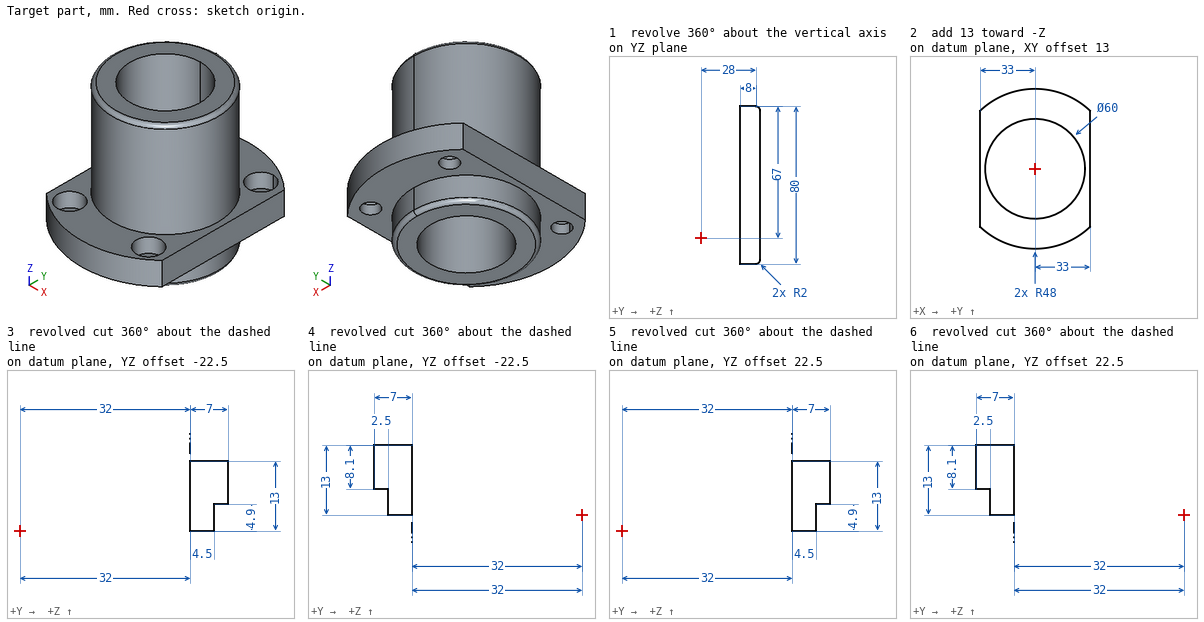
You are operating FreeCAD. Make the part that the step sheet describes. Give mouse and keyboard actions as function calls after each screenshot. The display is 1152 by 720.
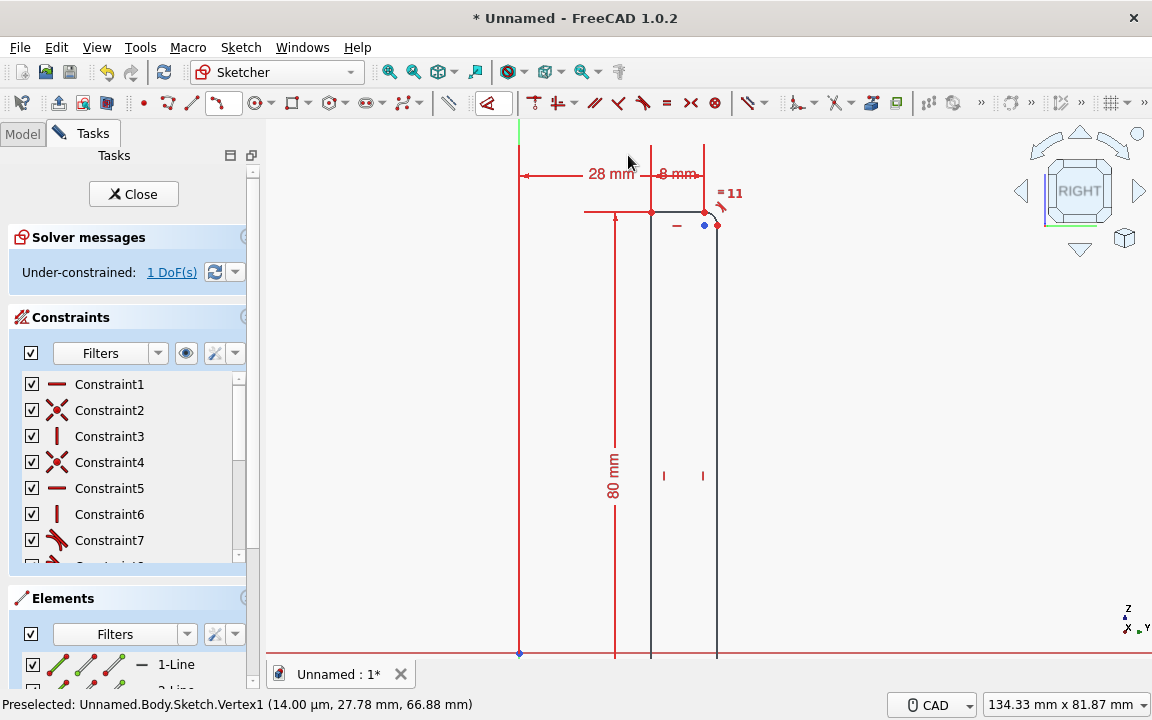
click(704, 212)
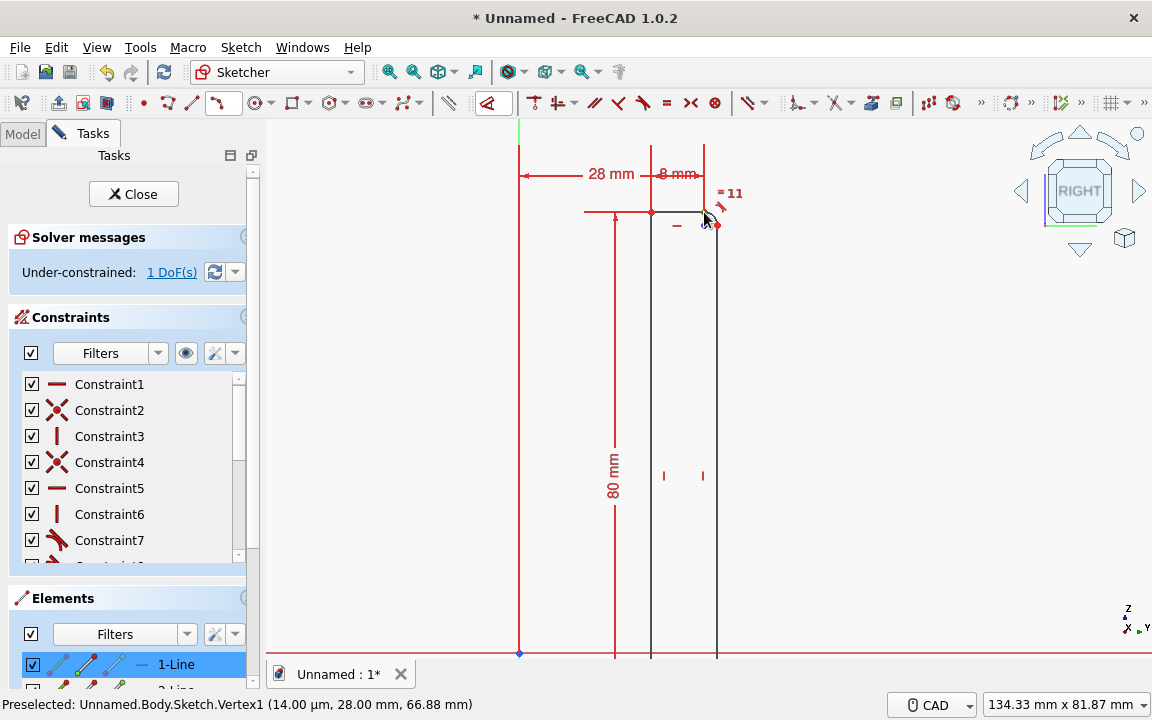
click(506, 104)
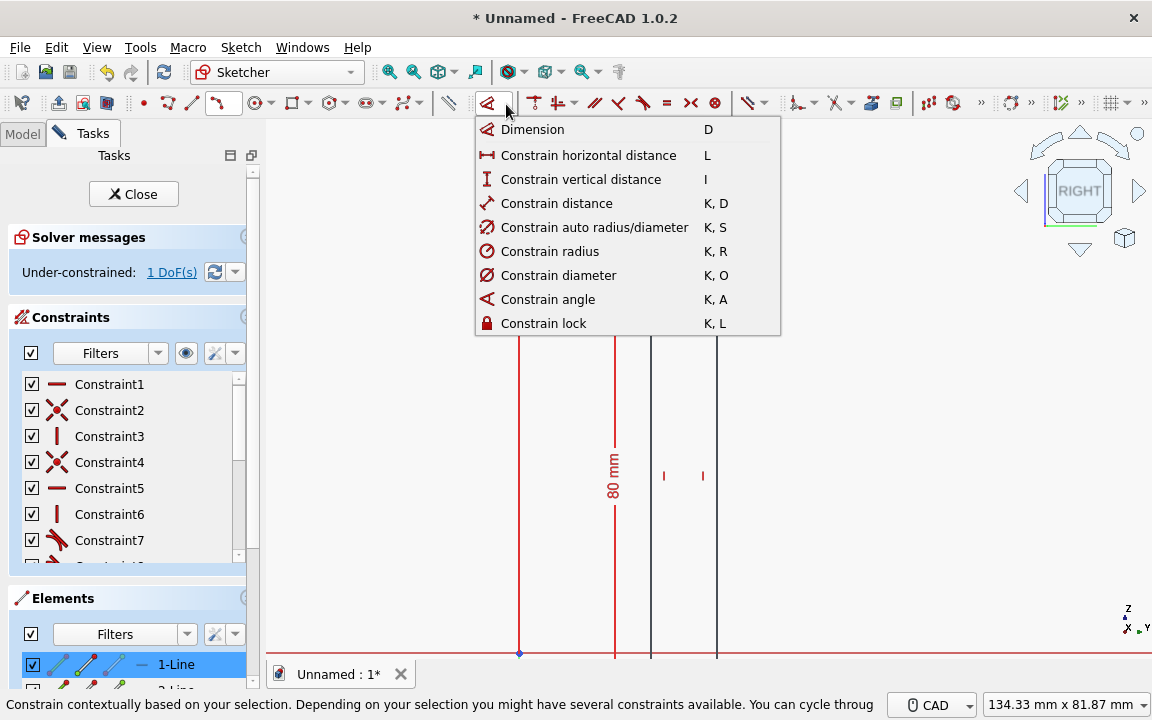
click(628, 179)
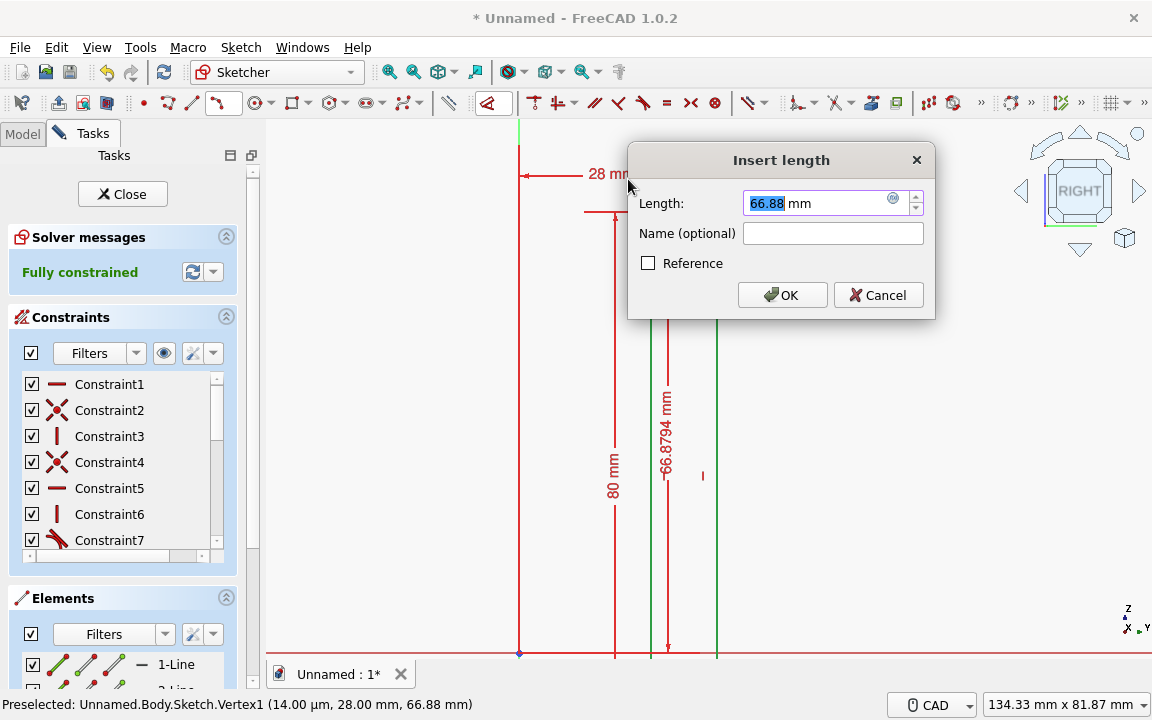
text(67)
key(Return)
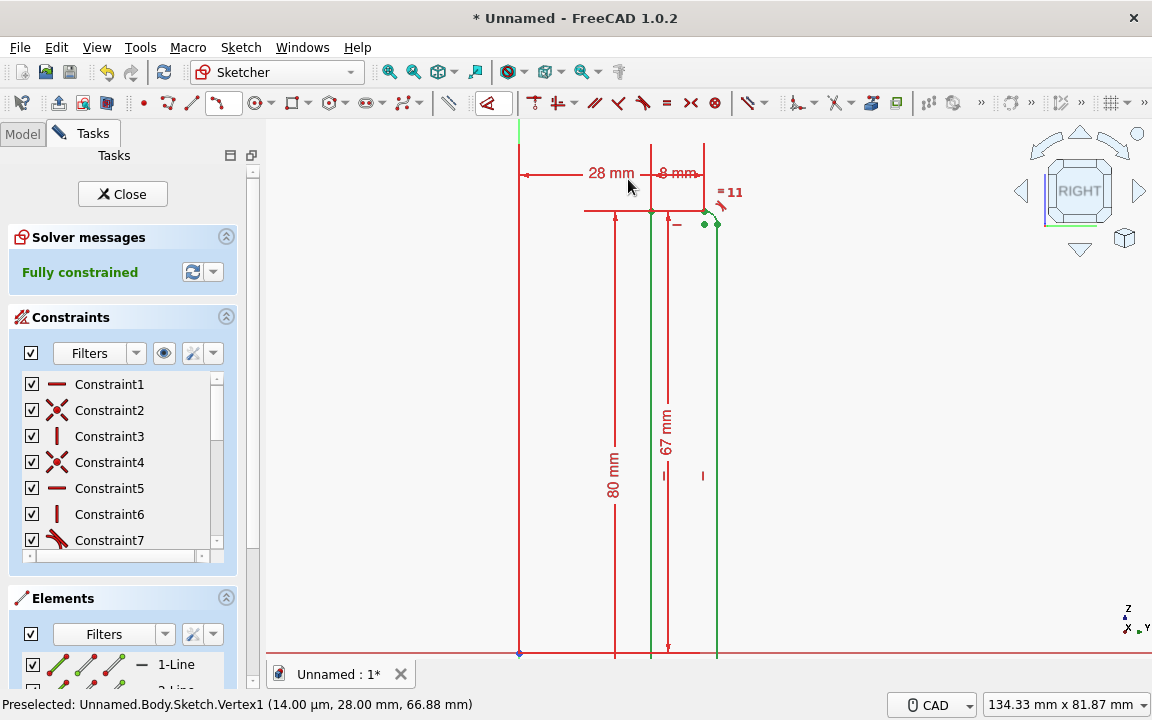
click(123, 194)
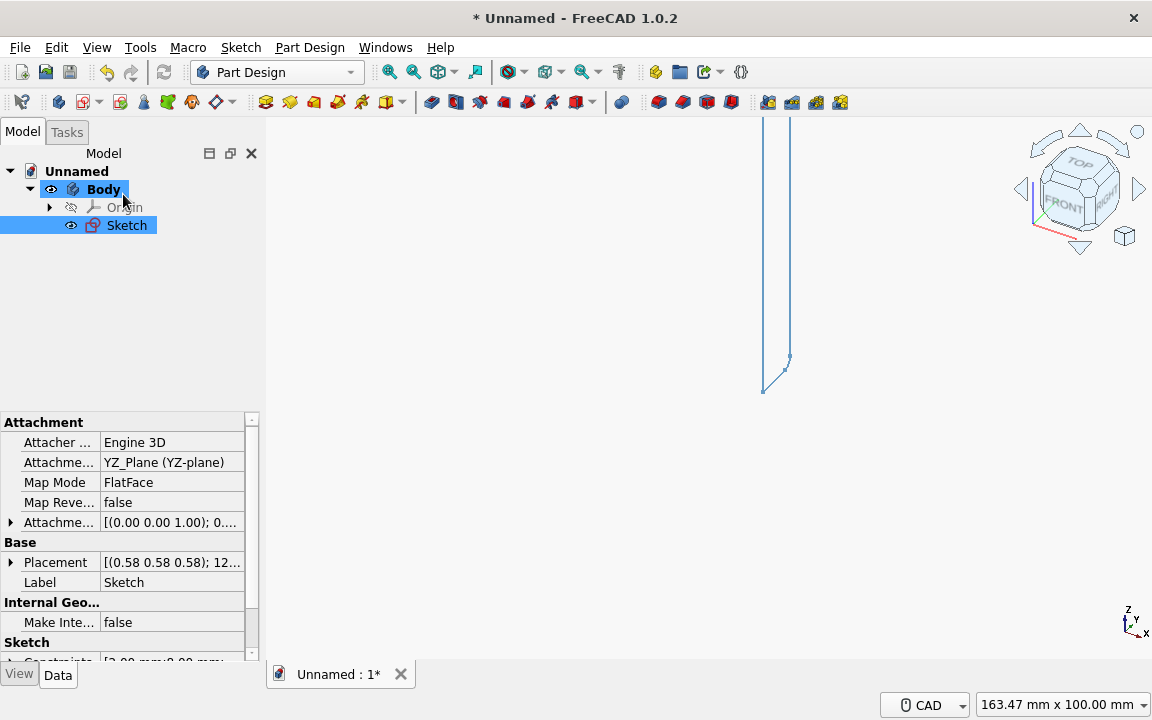
click(290, 102)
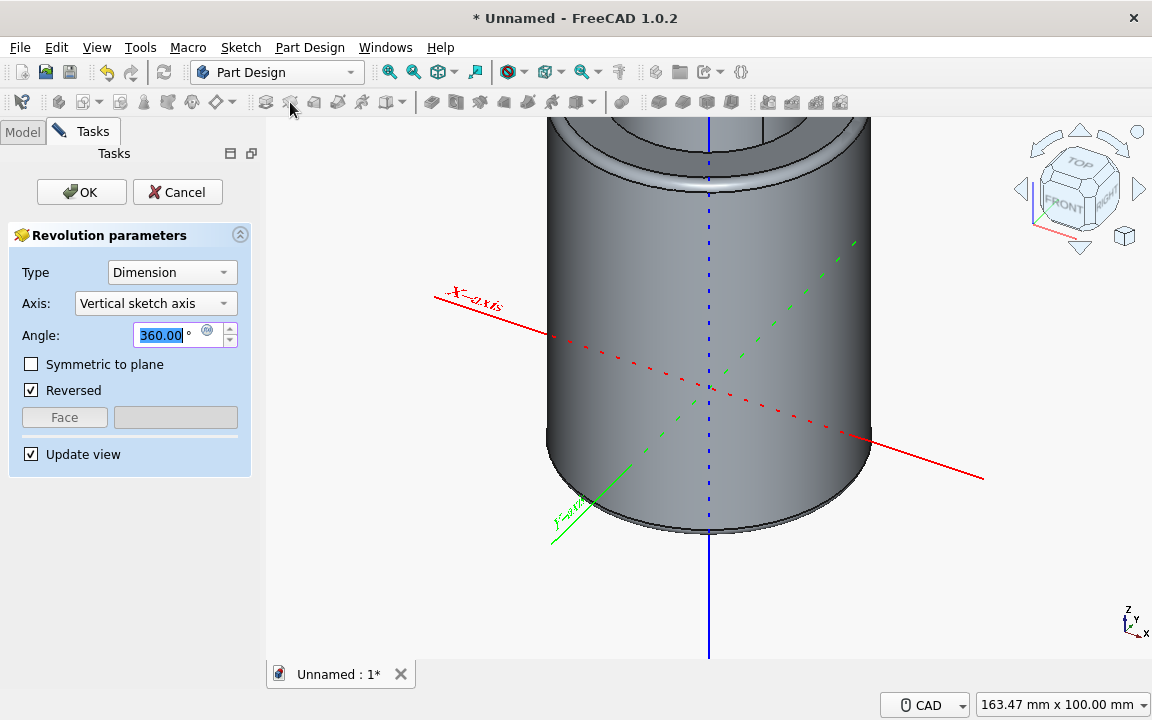
click(82, 192)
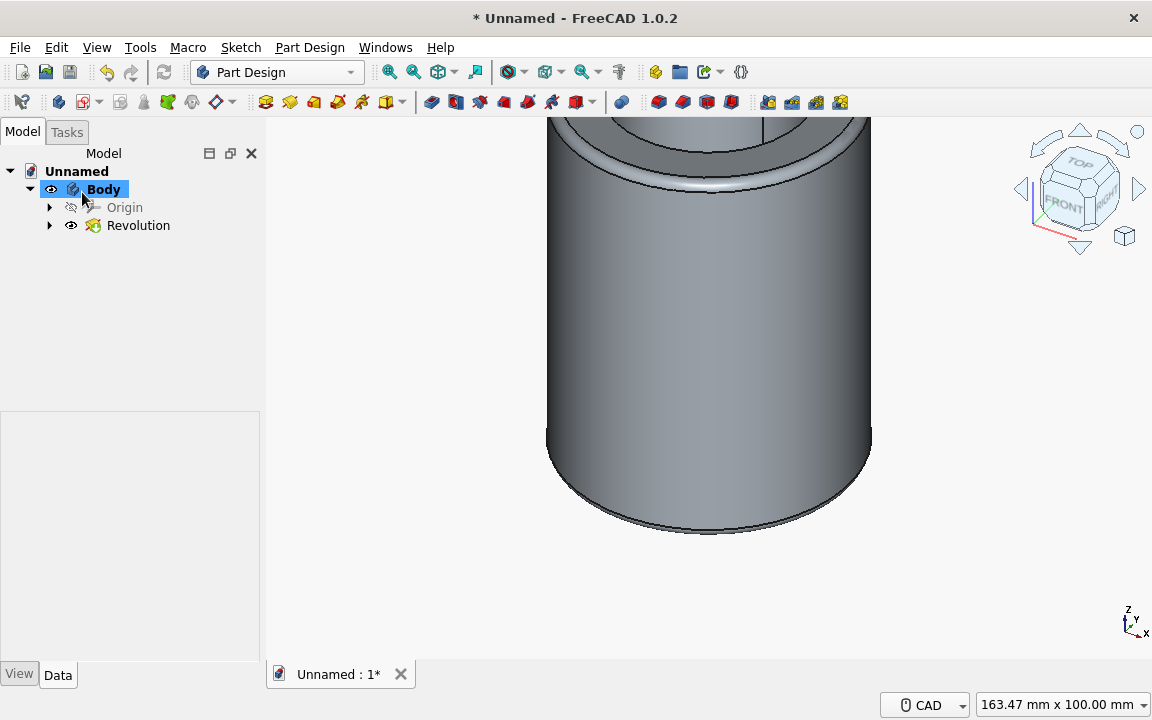
click(390, 72)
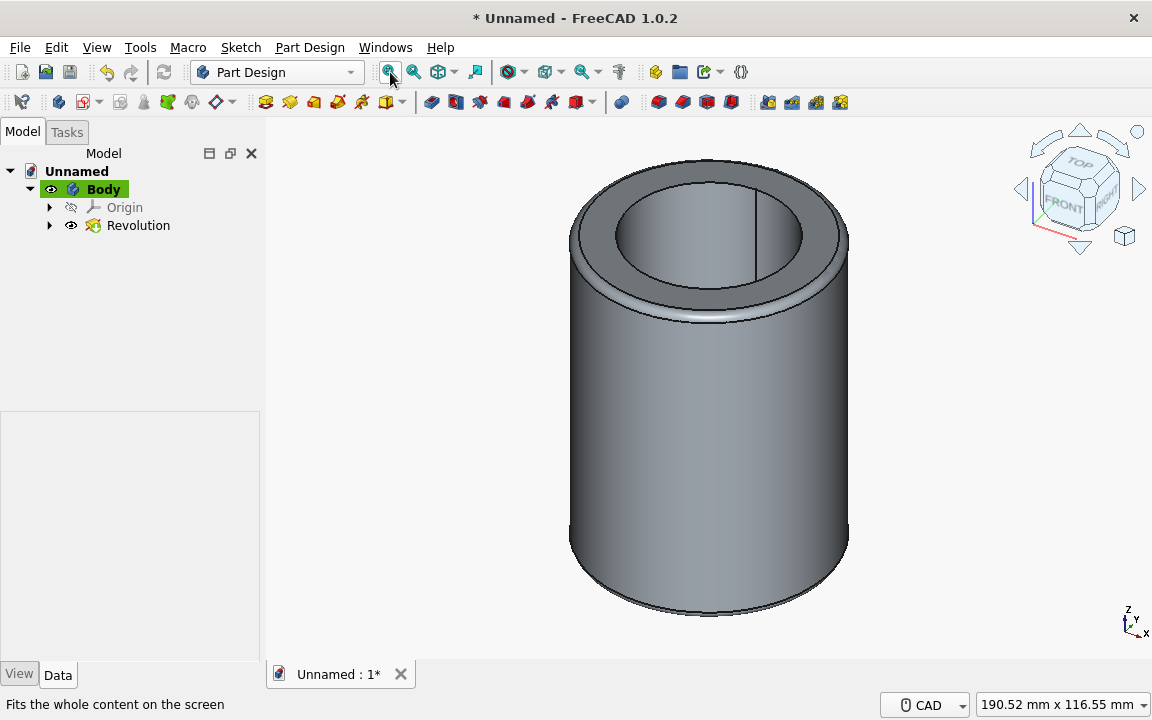
click(50, 207)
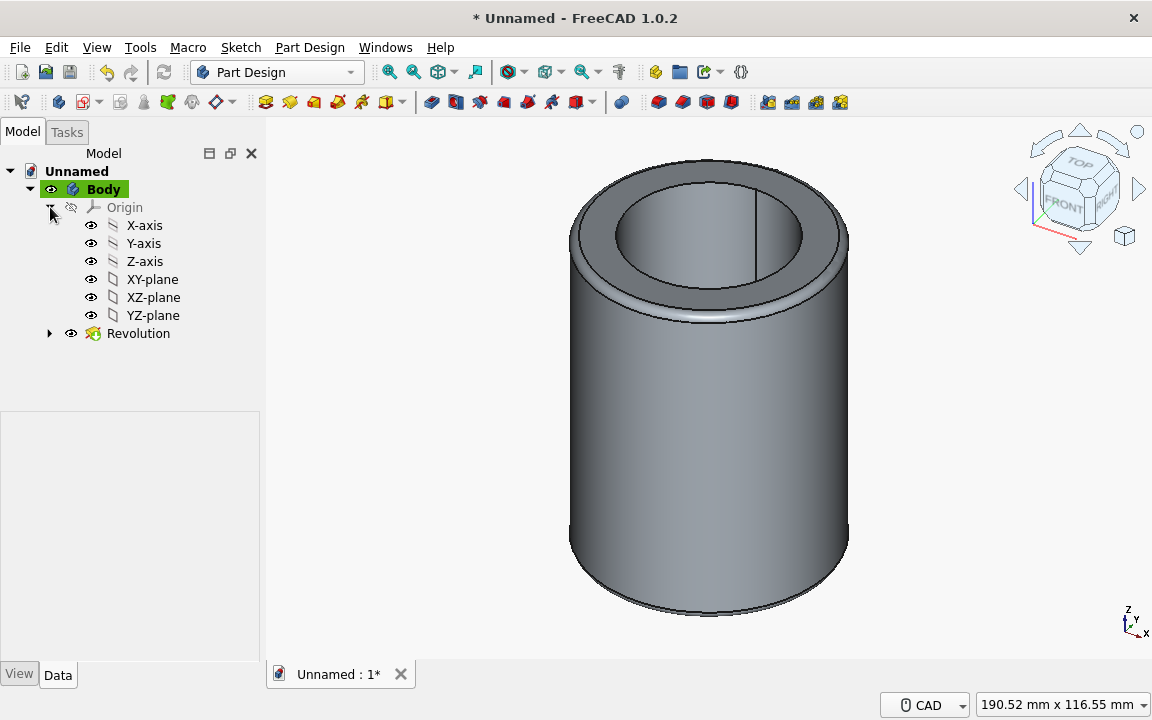
click(136, 279)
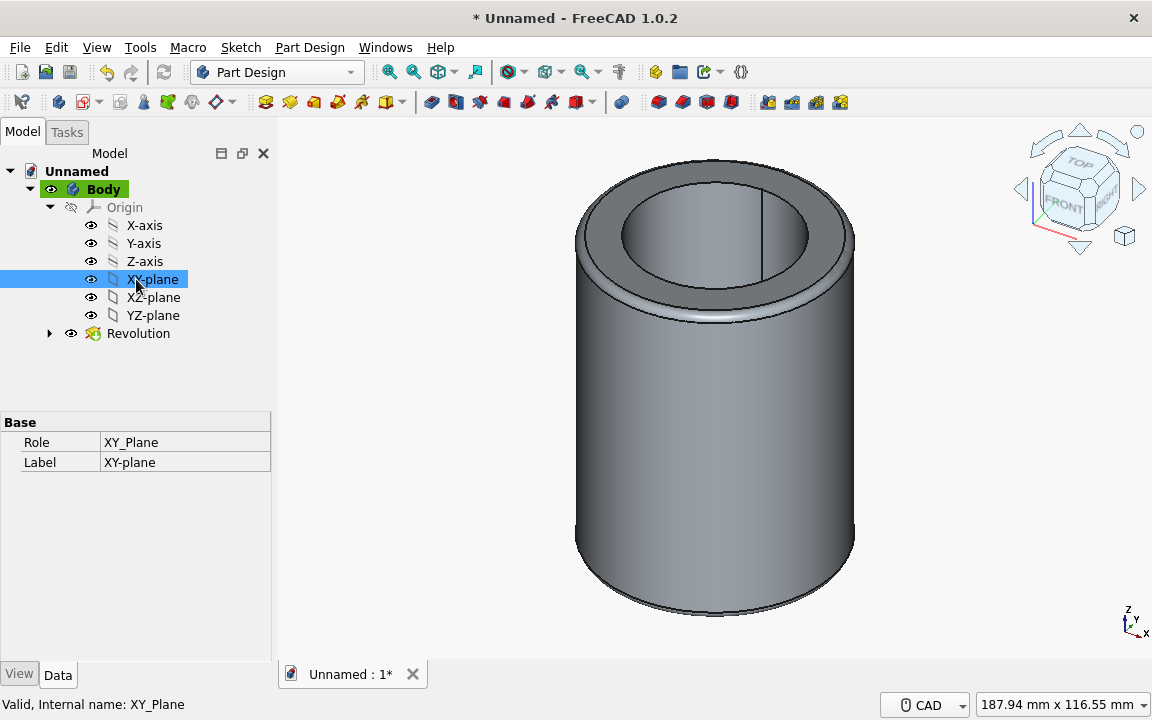
click(216, 102)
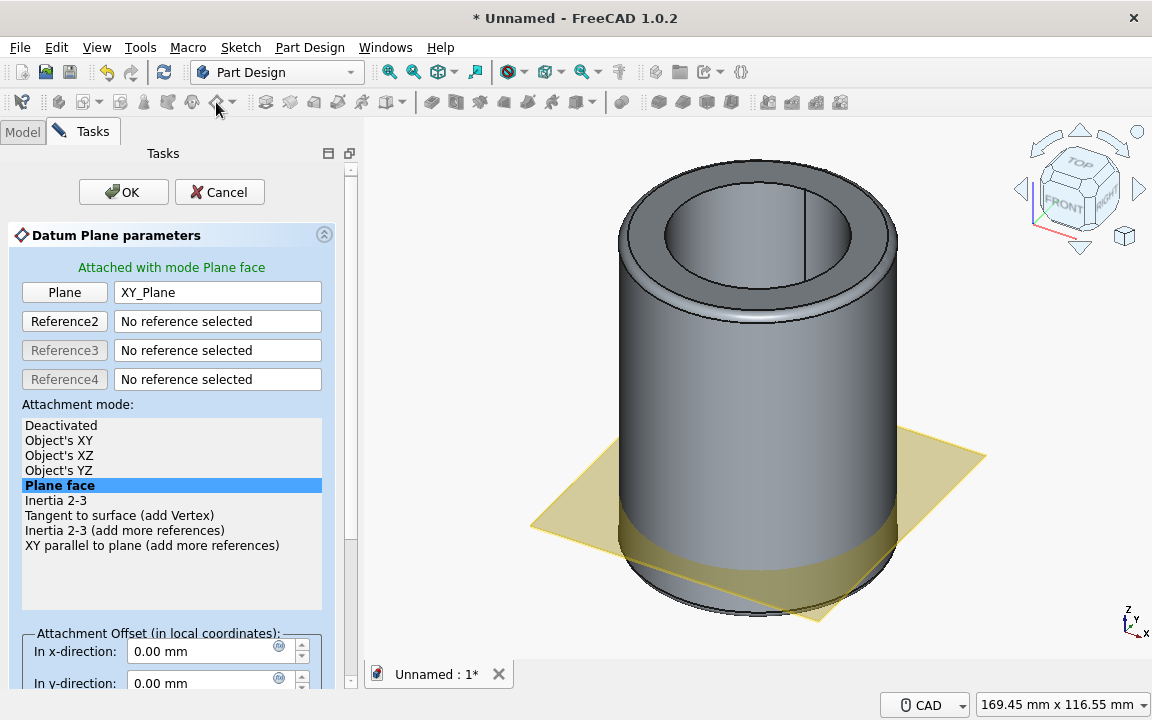
scroll(351, 426, down, 2)